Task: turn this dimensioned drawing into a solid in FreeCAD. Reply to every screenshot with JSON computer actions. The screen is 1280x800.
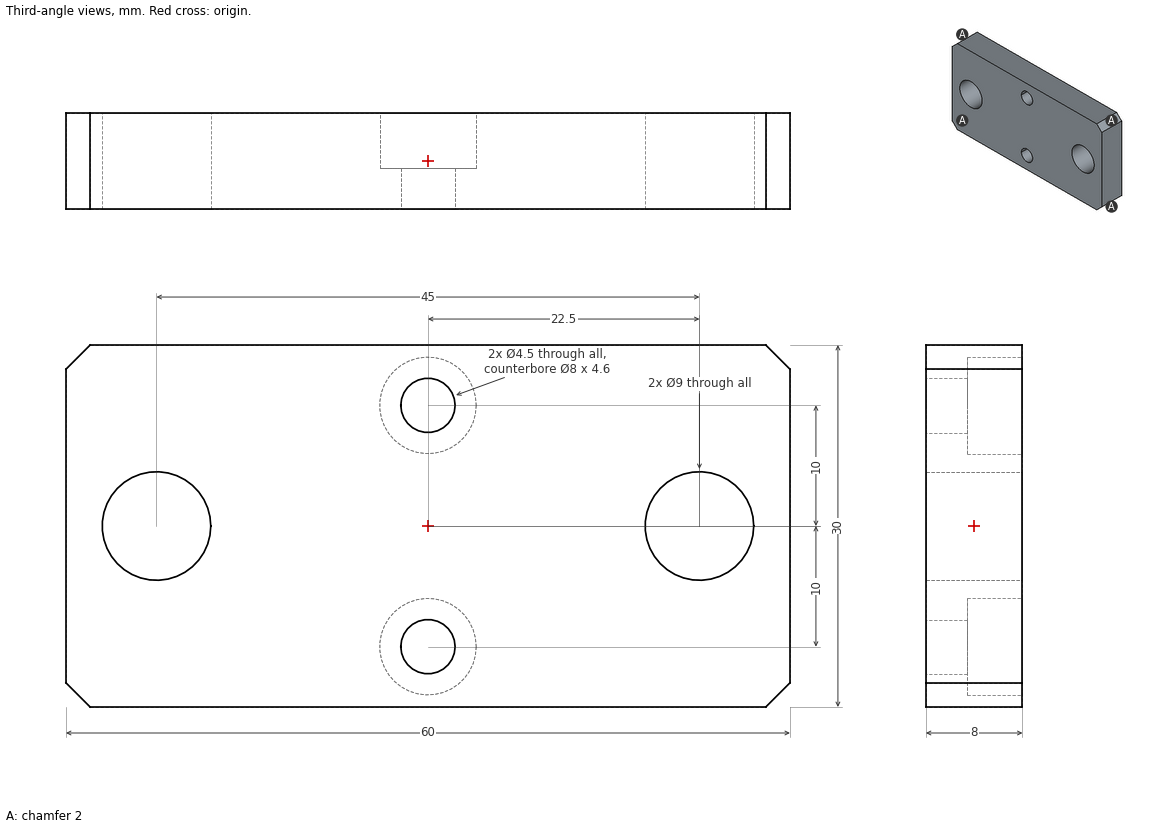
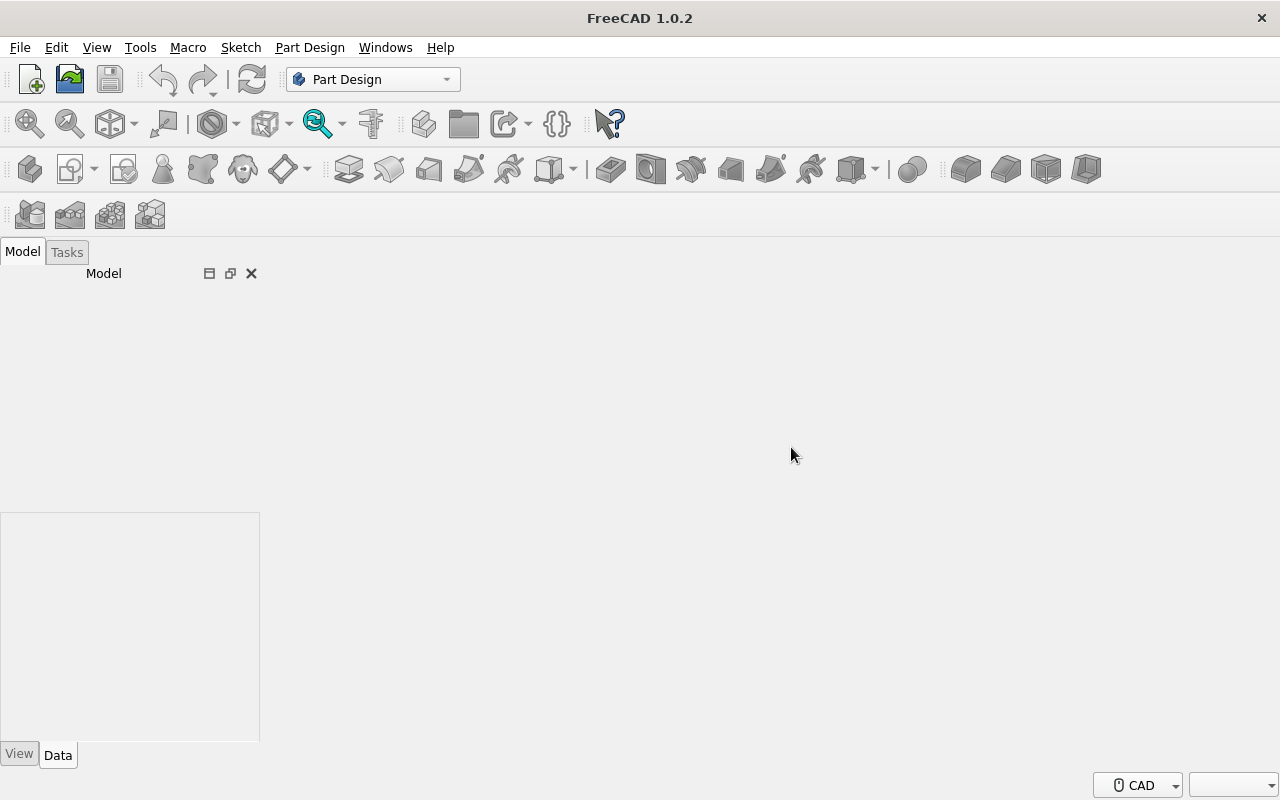
{"action": "left_click", "coordinate": [30, 80]}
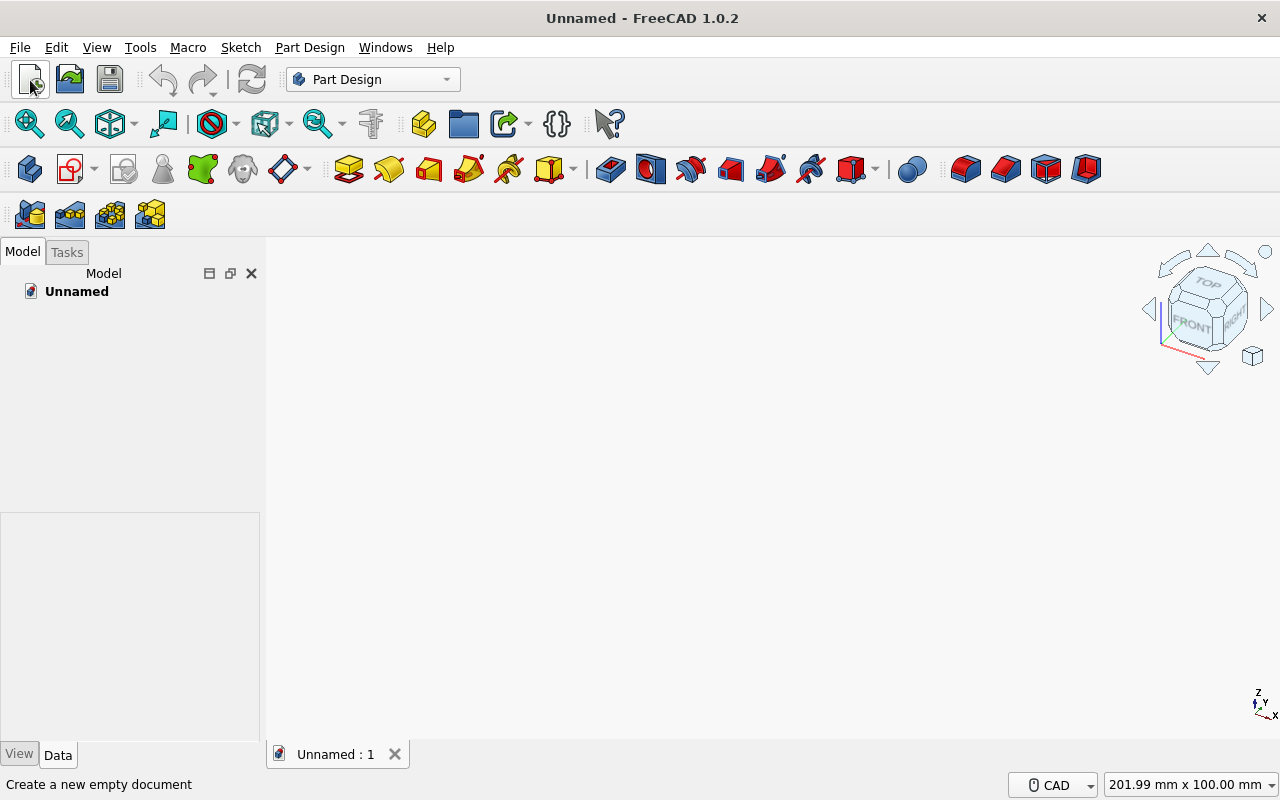
{"action": "left_click", "coordinate": [70, 170]}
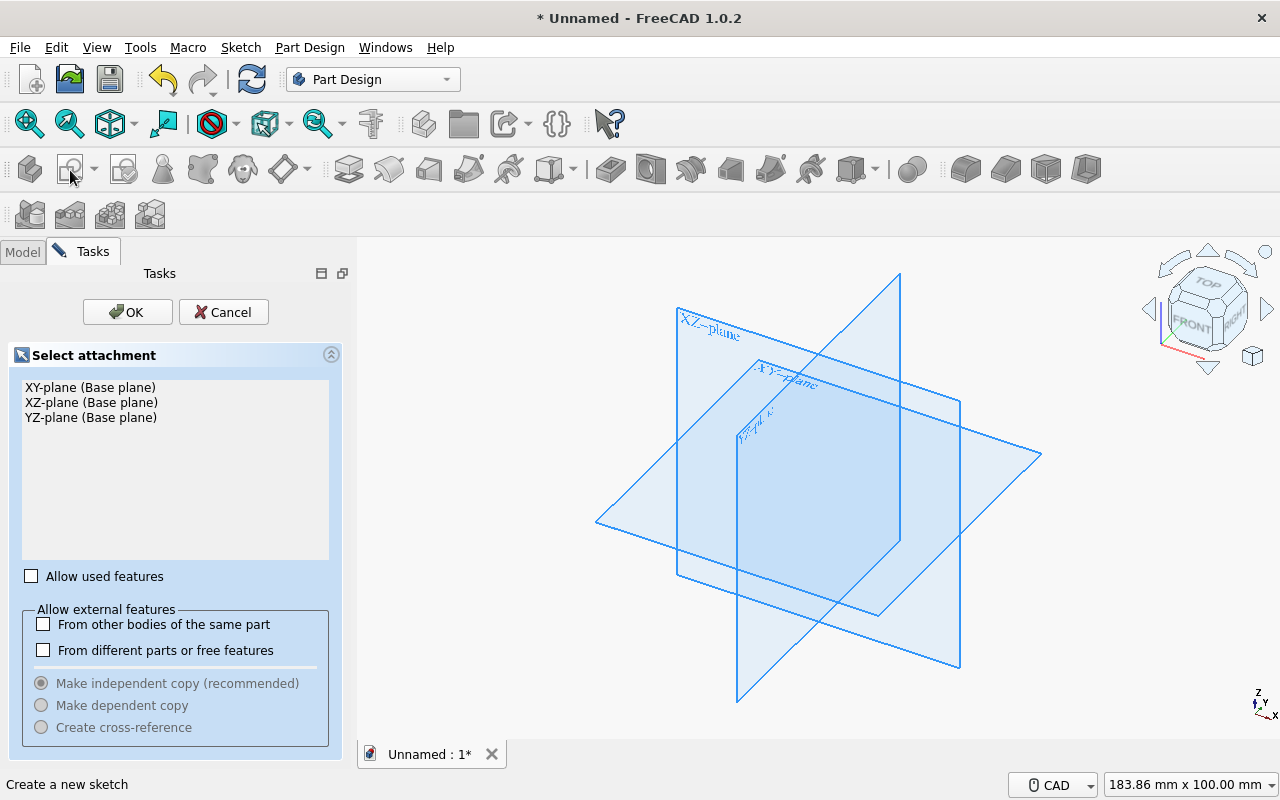
{"action": "left_click", "coordinate": [82, 402]}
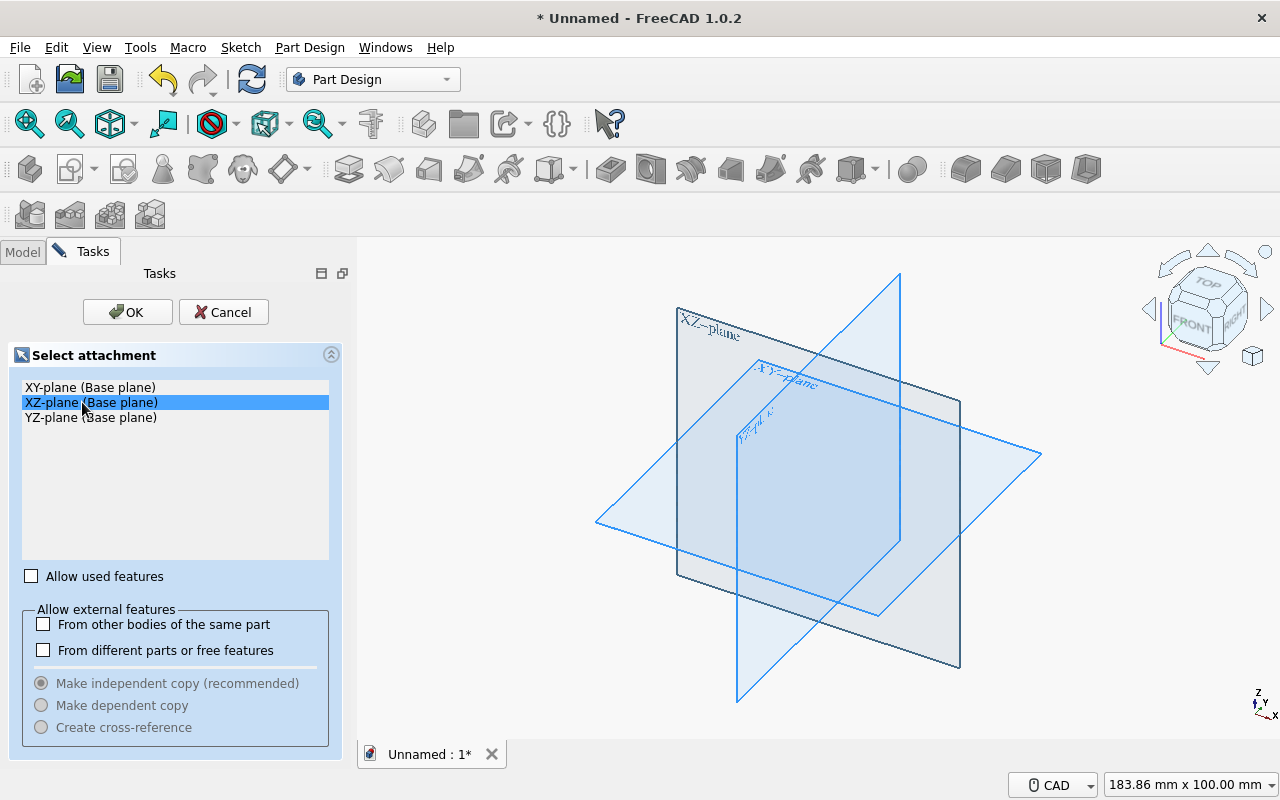
{"action": "left_click", "coordinate": [128, 312]}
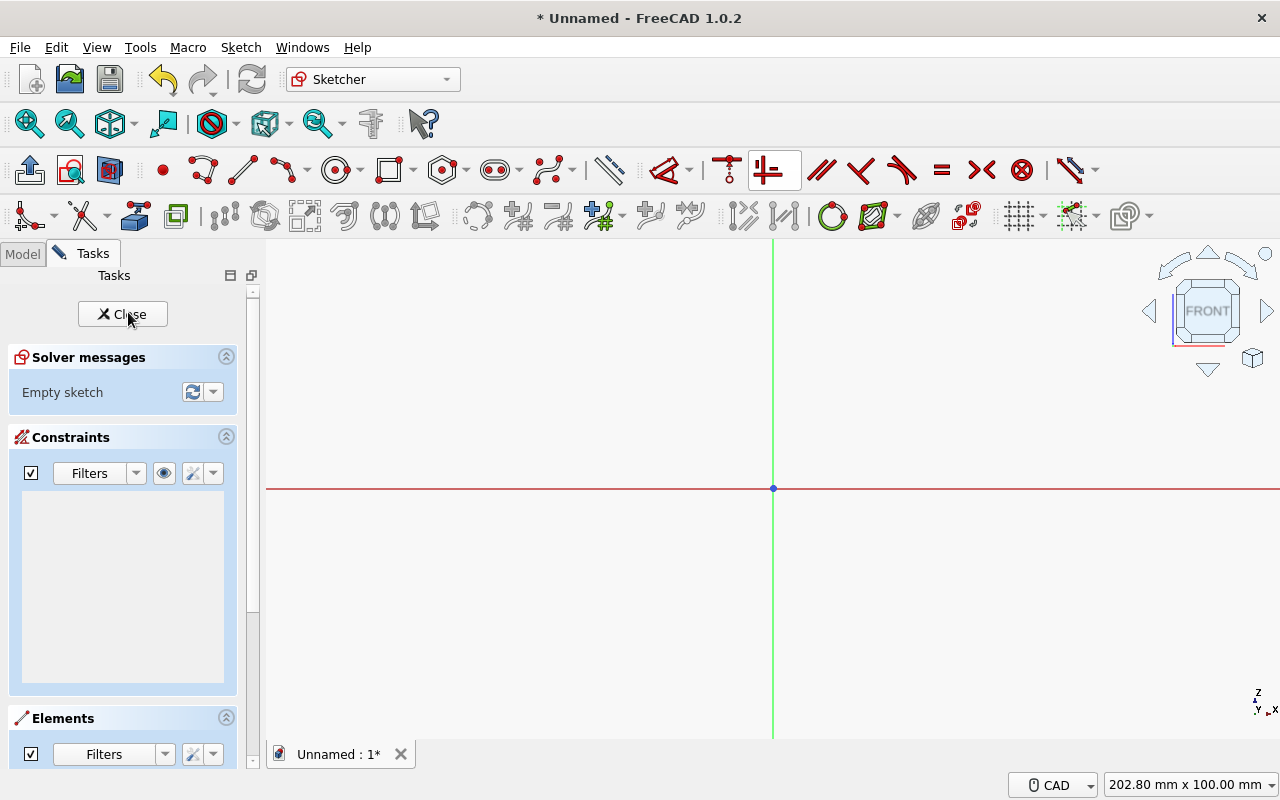
{"action": "scroll", "coordinate": [856, 489], "scroll_direction": "up", "scroll_amount": 3}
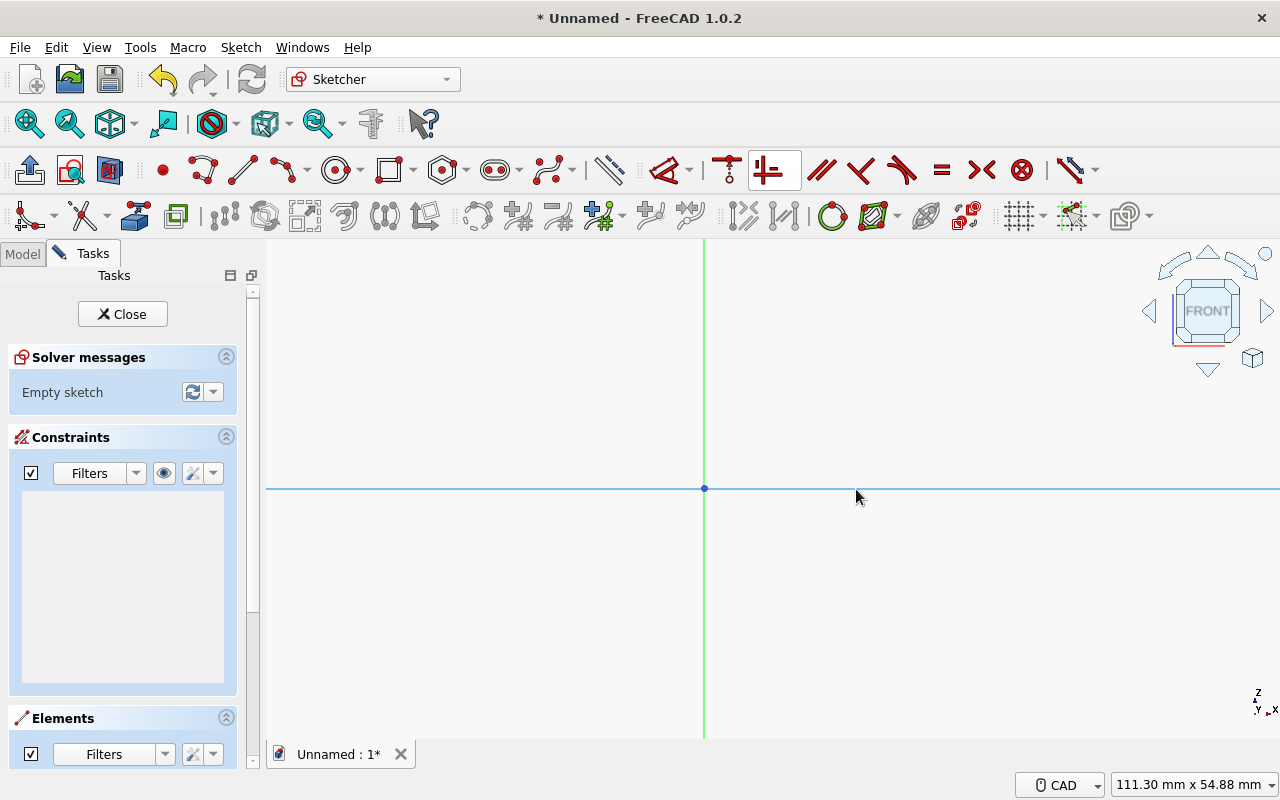
{"action": "key", "text": "g v"}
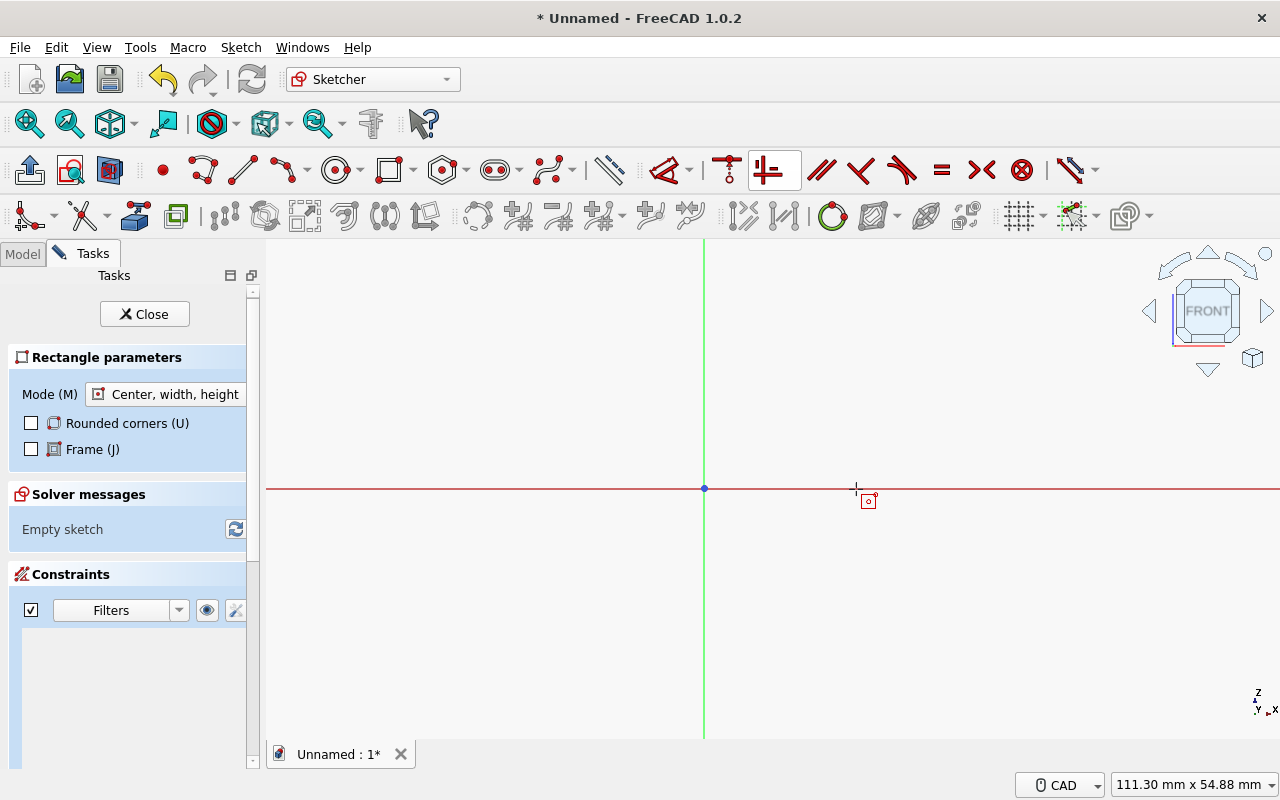
{"action": "left_click", "coordinate": [704, 489]}
{"action": "left_click", "coordinate": [978, 352]}
{"action": "key", "text": "Escape"}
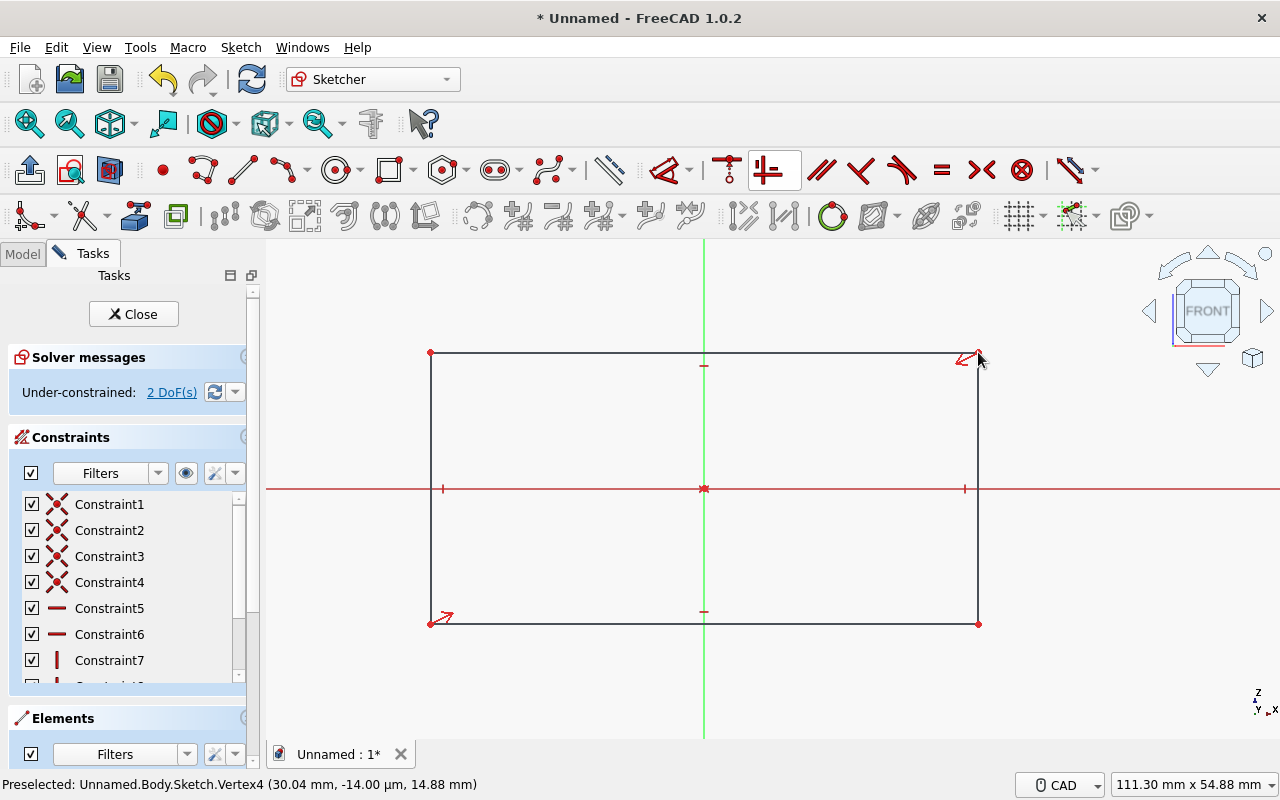
{"action": "left_click", "coordinate": [595, 624]}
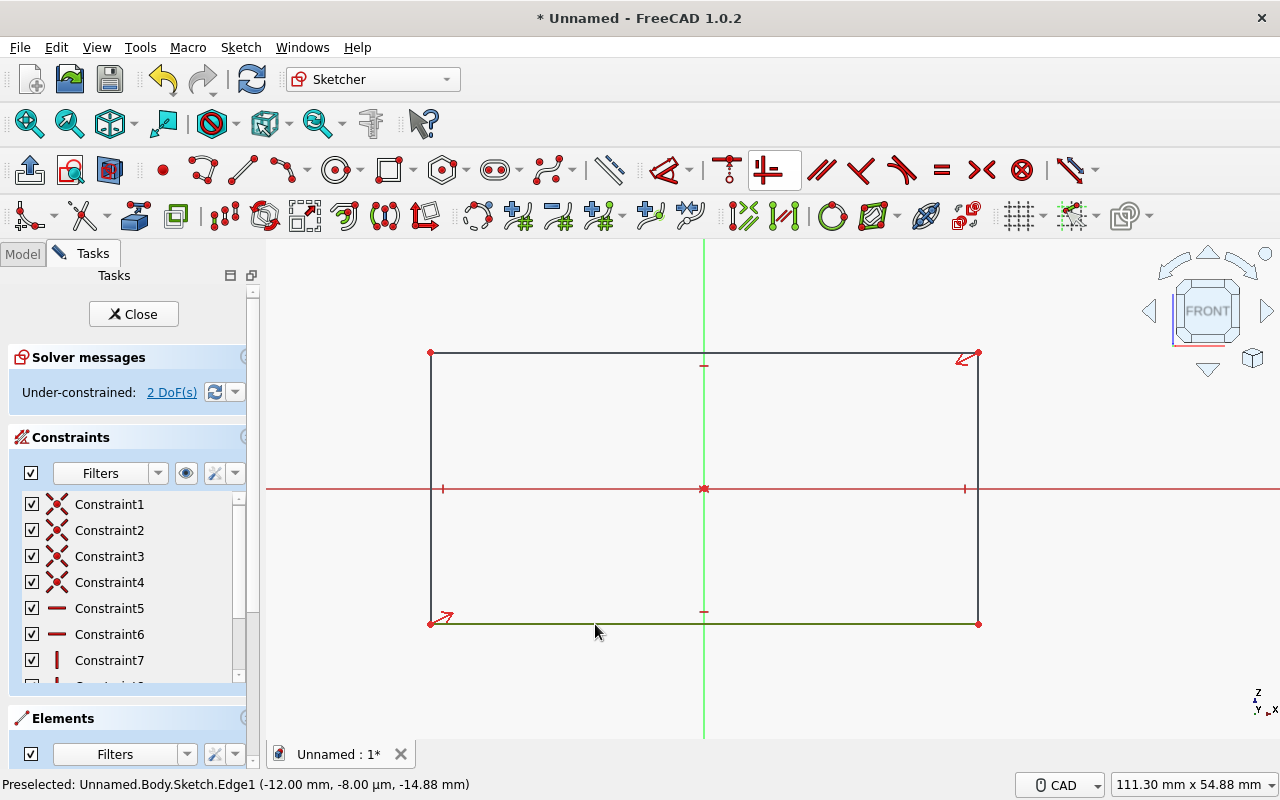
{"action": "left_click", "coordinate": [692, 170]}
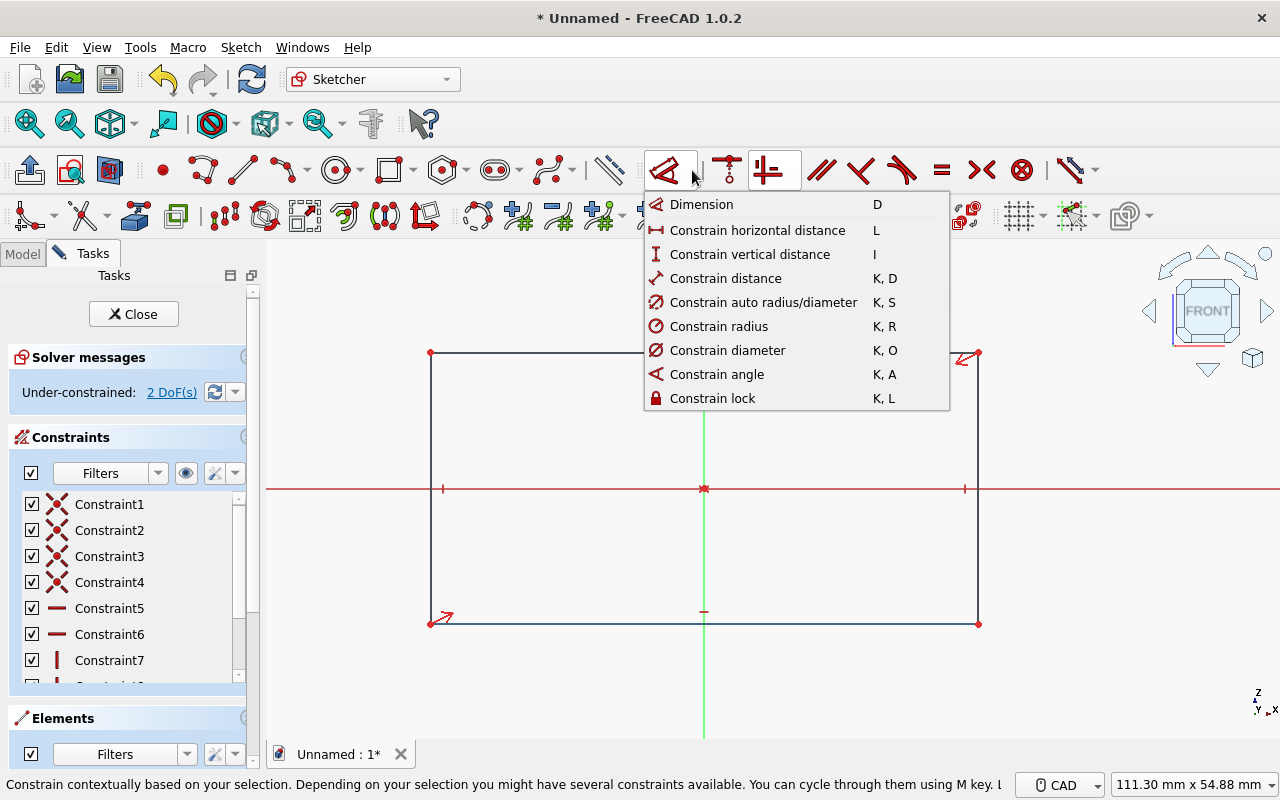
{"action": "left_click", "coordinate": [797, 230]}